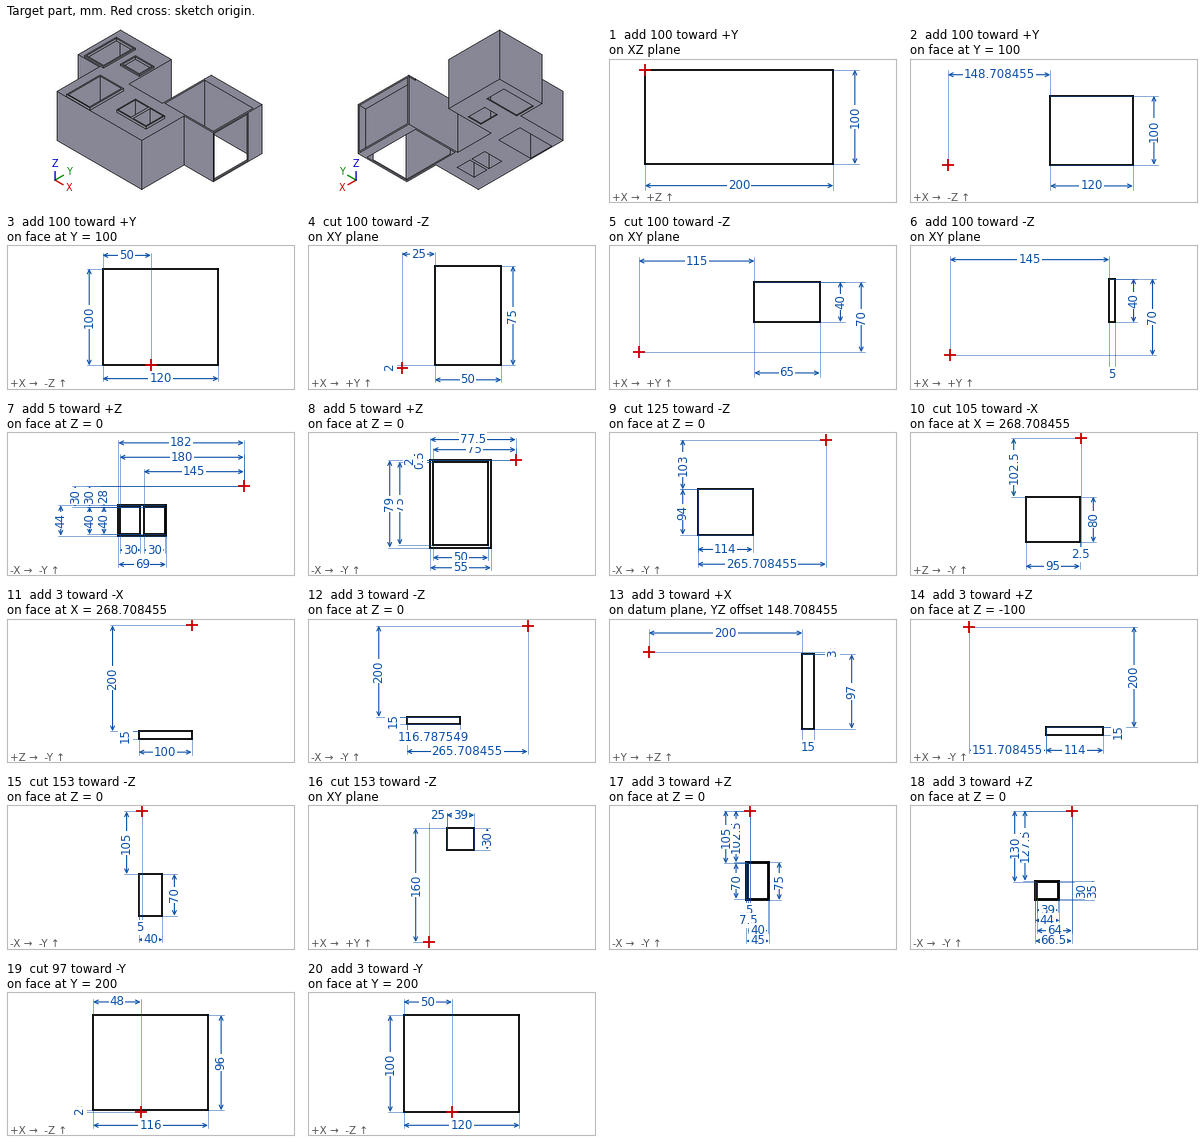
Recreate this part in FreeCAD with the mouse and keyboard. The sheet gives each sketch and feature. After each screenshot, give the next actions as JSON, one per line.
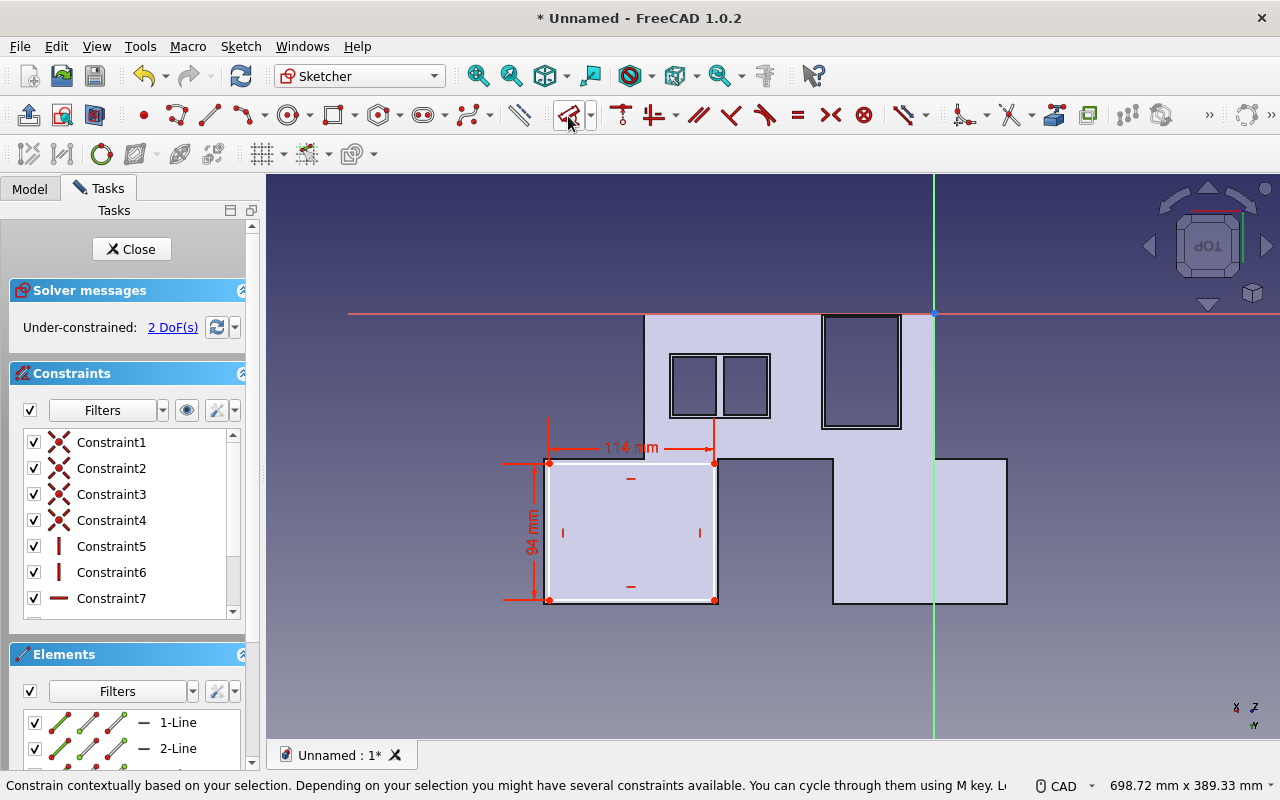
{"action": "left_click", "coordinate": [549, 464]}
{"action": "left_click", "coordinate": [968, 389]}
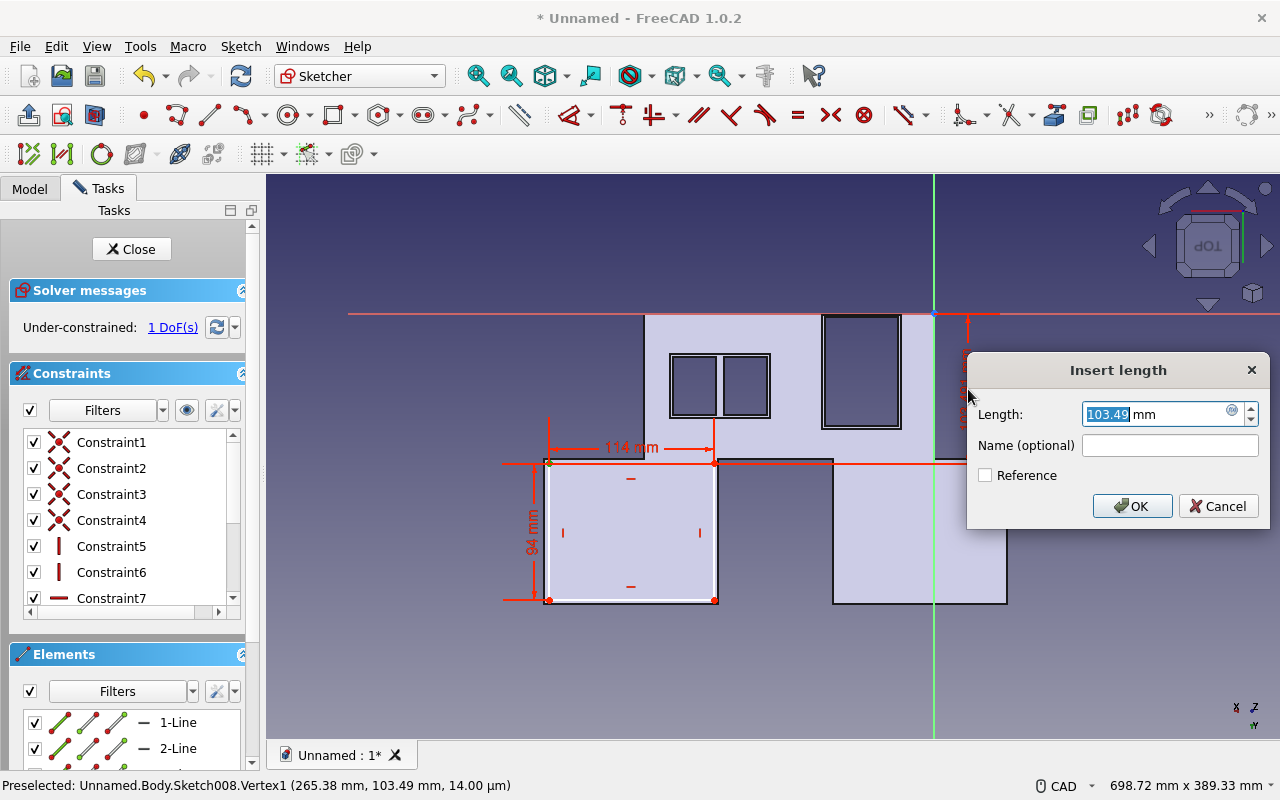
{"action": "type", "text": "103"}
{"action": "key", "text": "Return"}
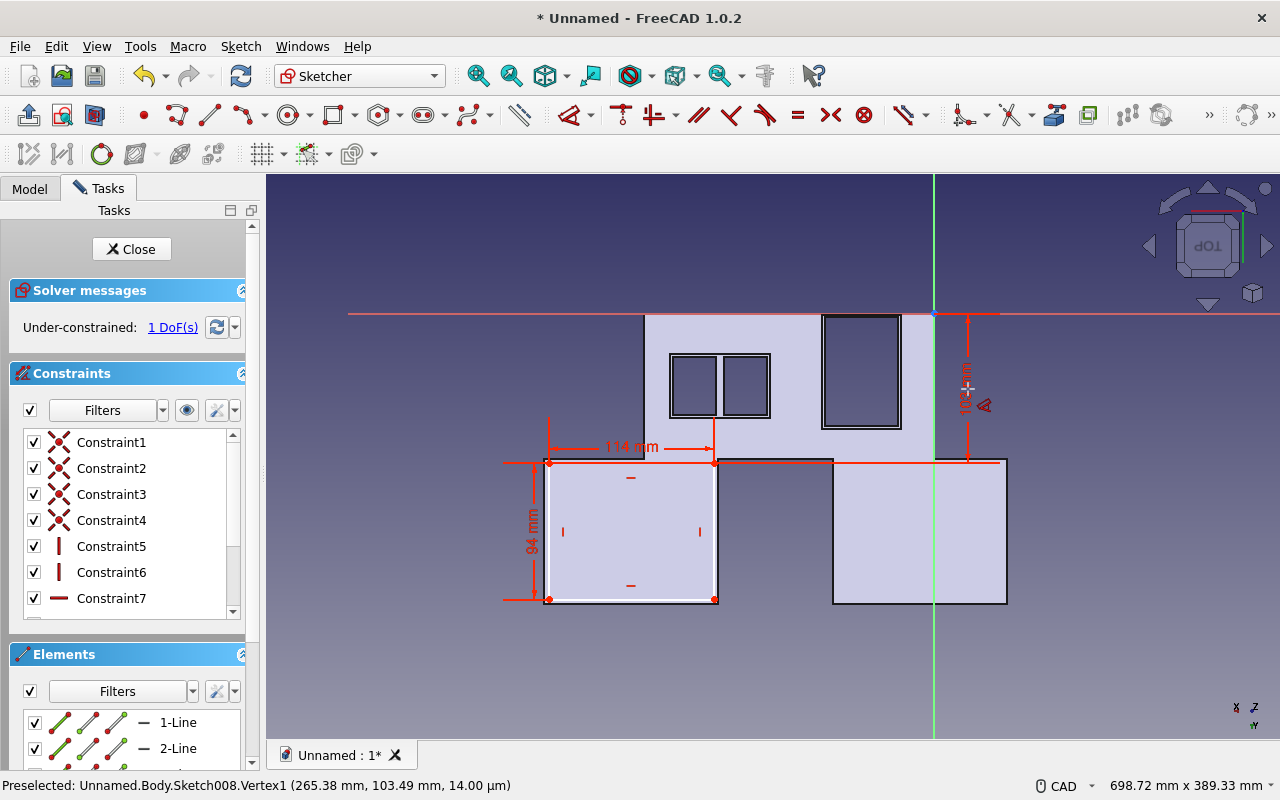
{"action": "left_click", "coordinate": [549, 463]}
{"action": "left_click", "coordinate": [742, 280]}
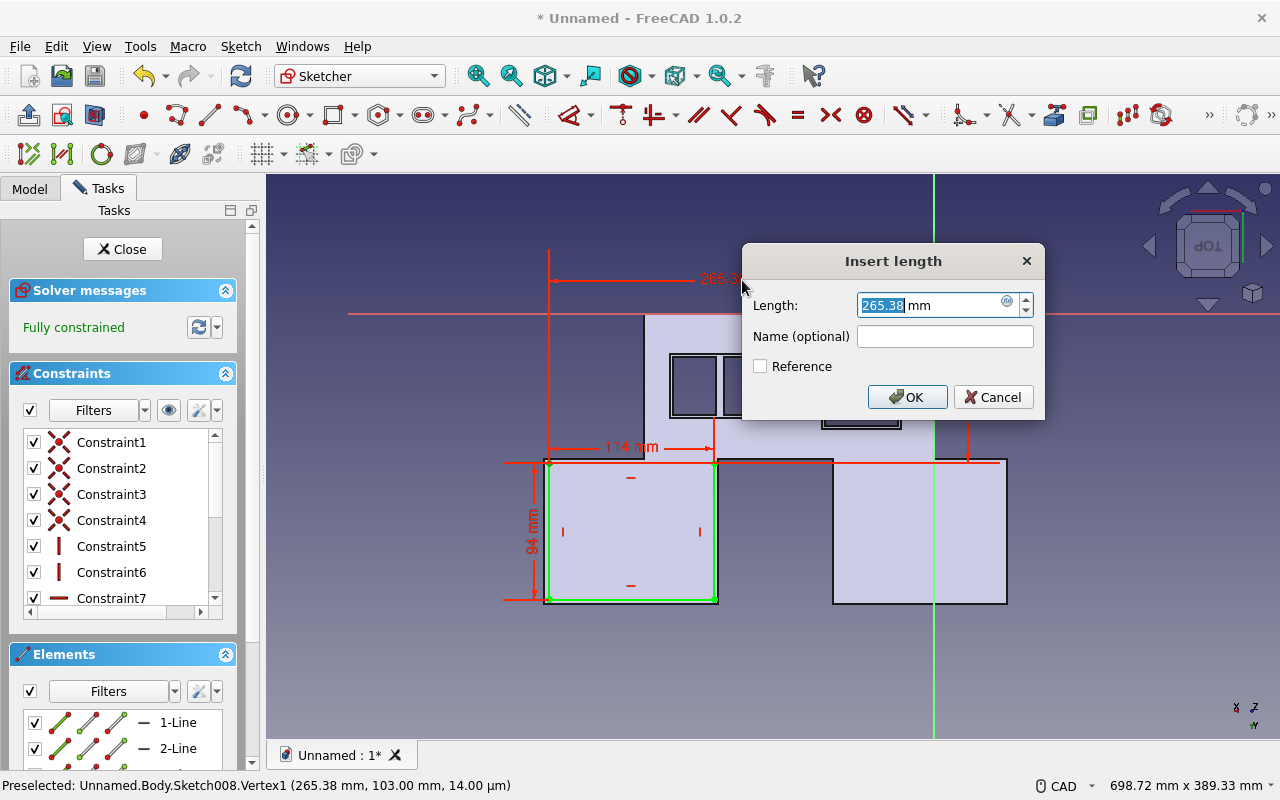
{"action": "type", "text": "265.708455"}
{"action": "key", "text": "Return"}
{"action": "key", "text": "Escape"}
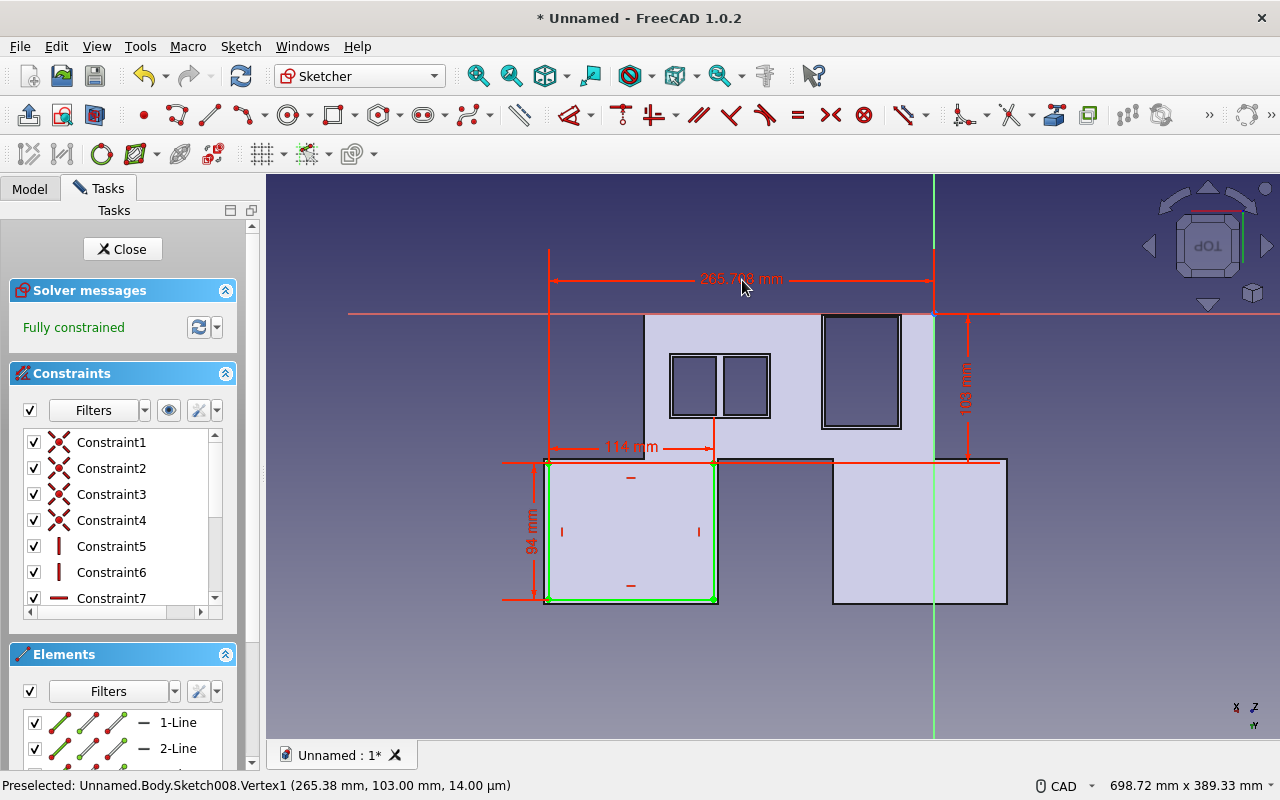
{"action": "left_click", "coordinate": [123, 249]}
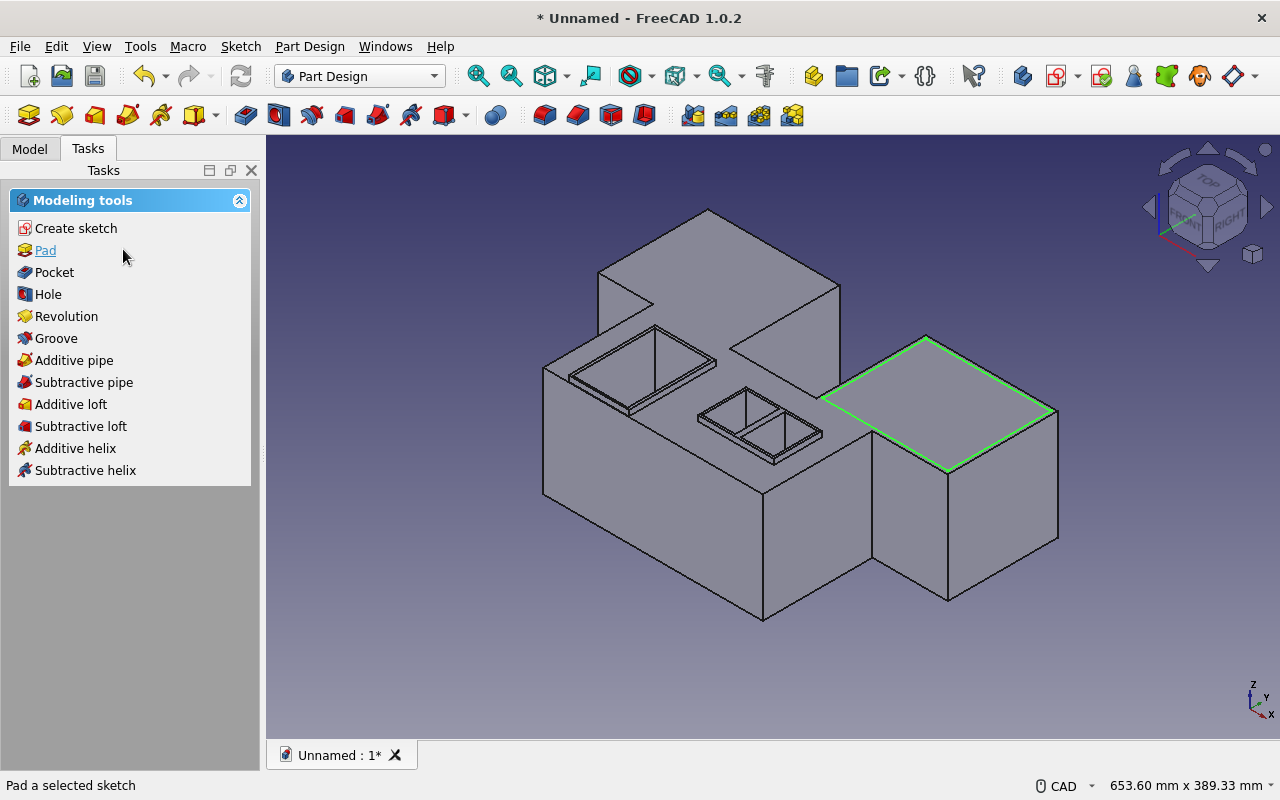
{"action": "left_click", "coordinate": [246, 116]}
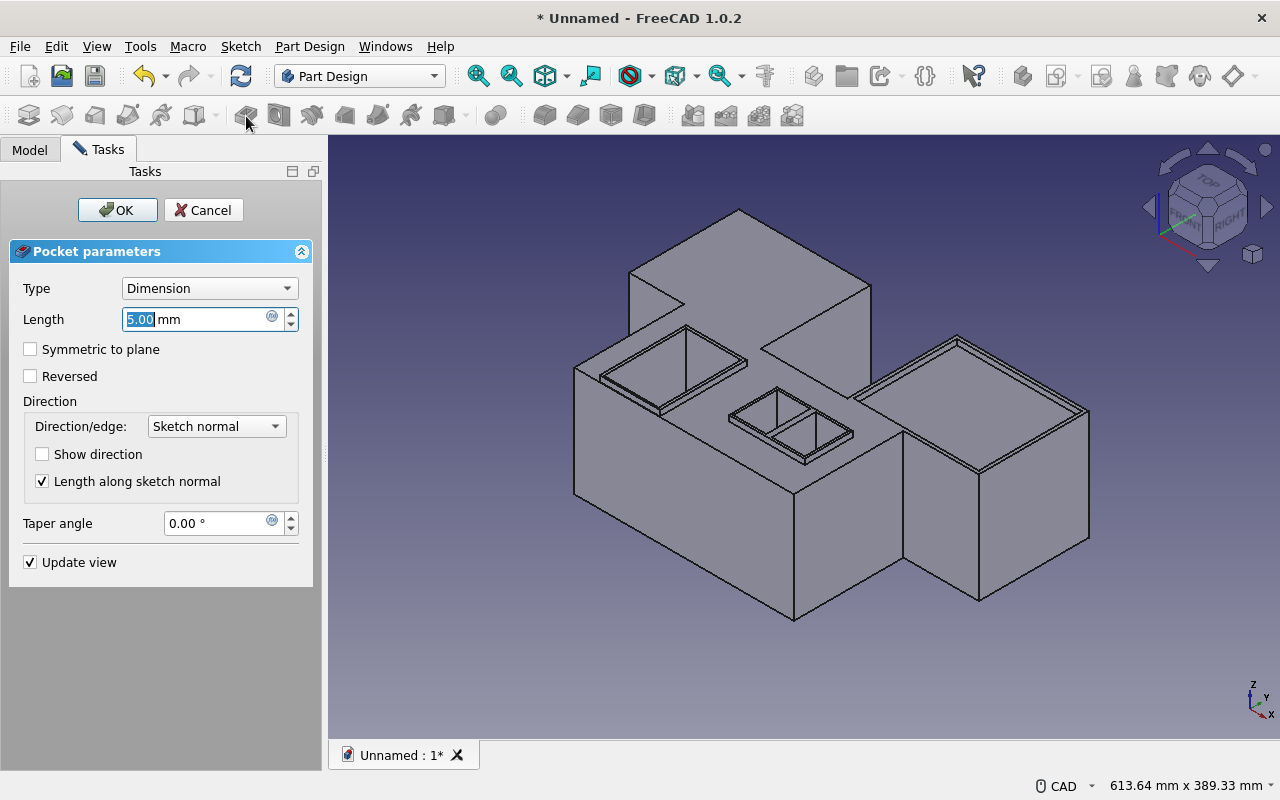
{"action": "type", "text": "125"}
{"action": "key", "text": "Tab"}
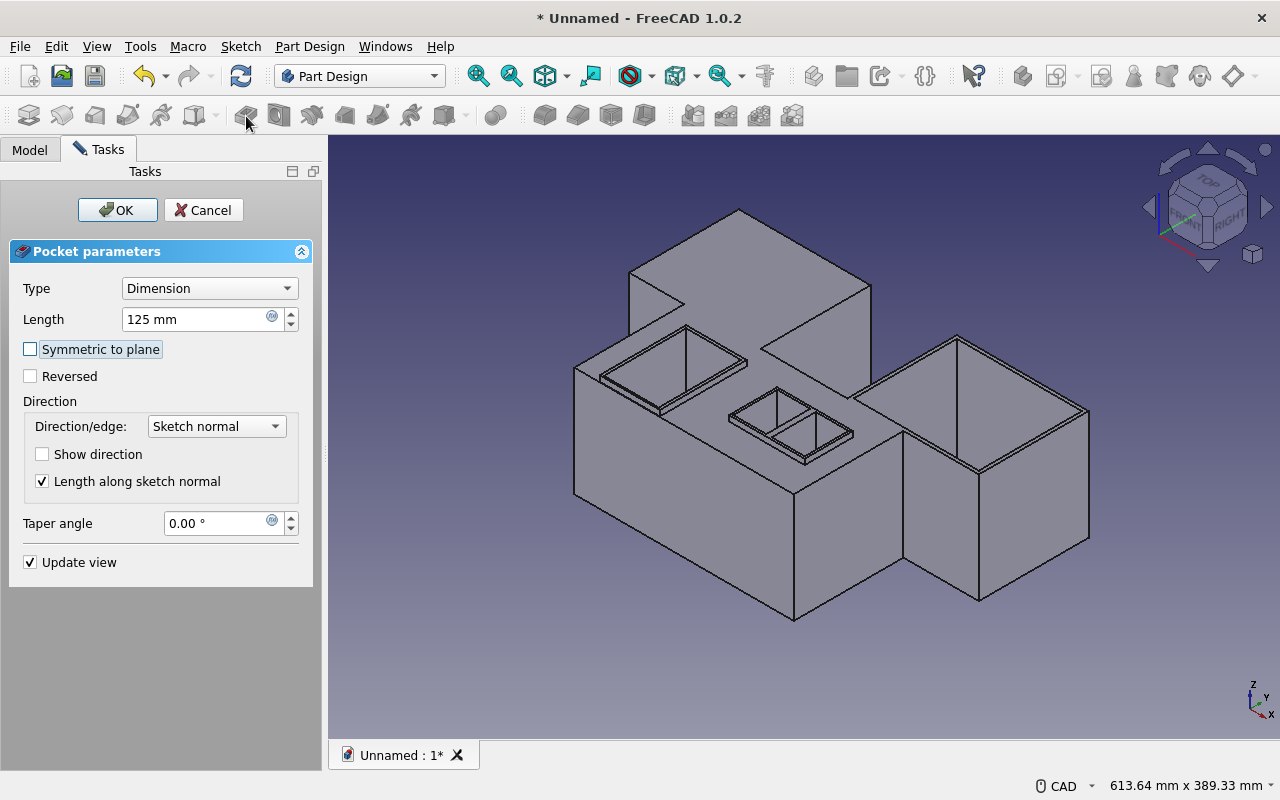
{"action": "left_click", "coordinate": [118, 210]}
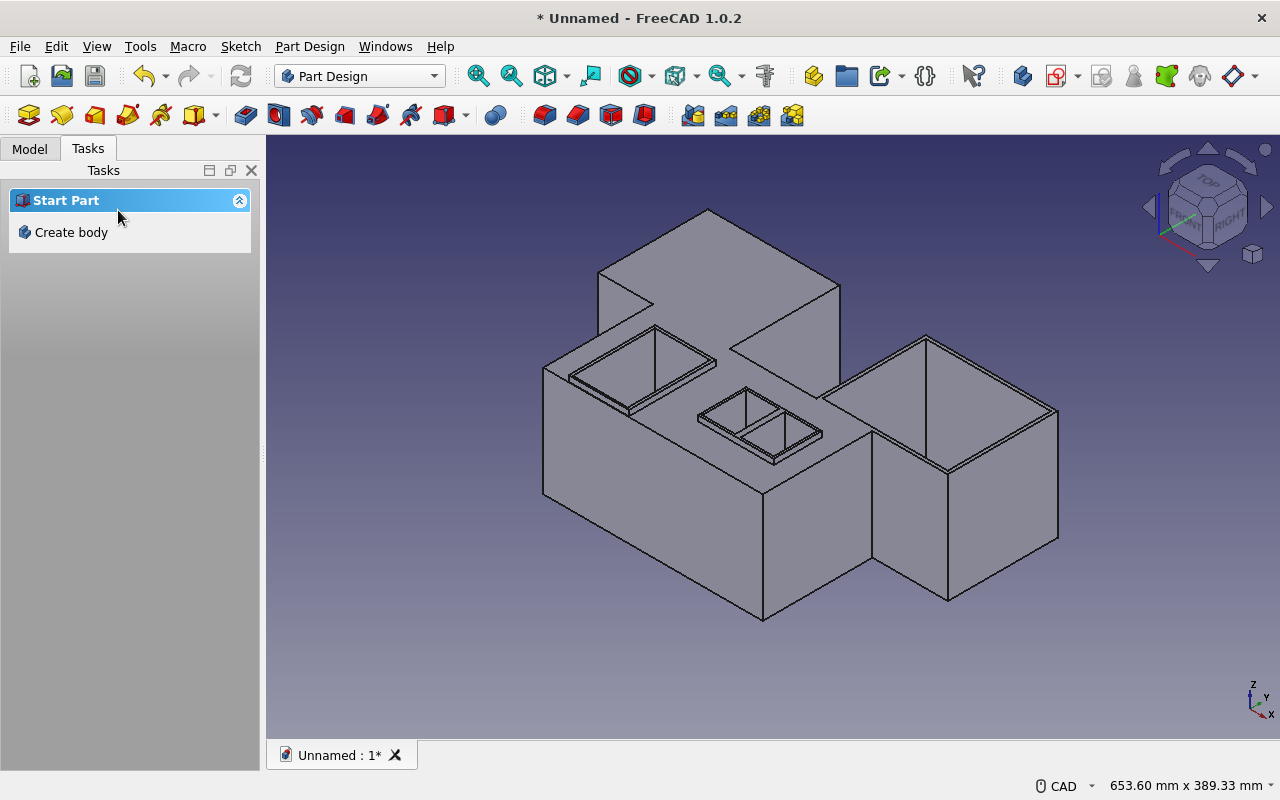
{"action": "left_click", "coordinate": [1003, 505]}